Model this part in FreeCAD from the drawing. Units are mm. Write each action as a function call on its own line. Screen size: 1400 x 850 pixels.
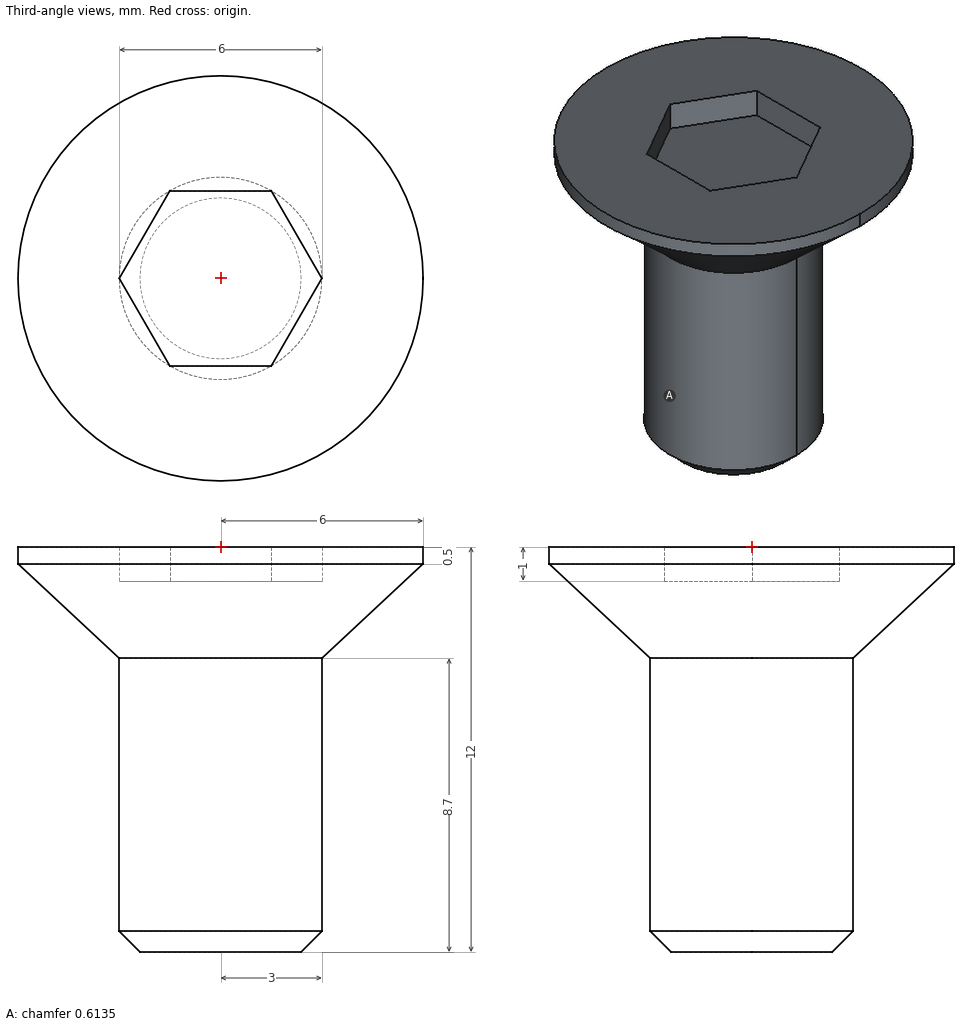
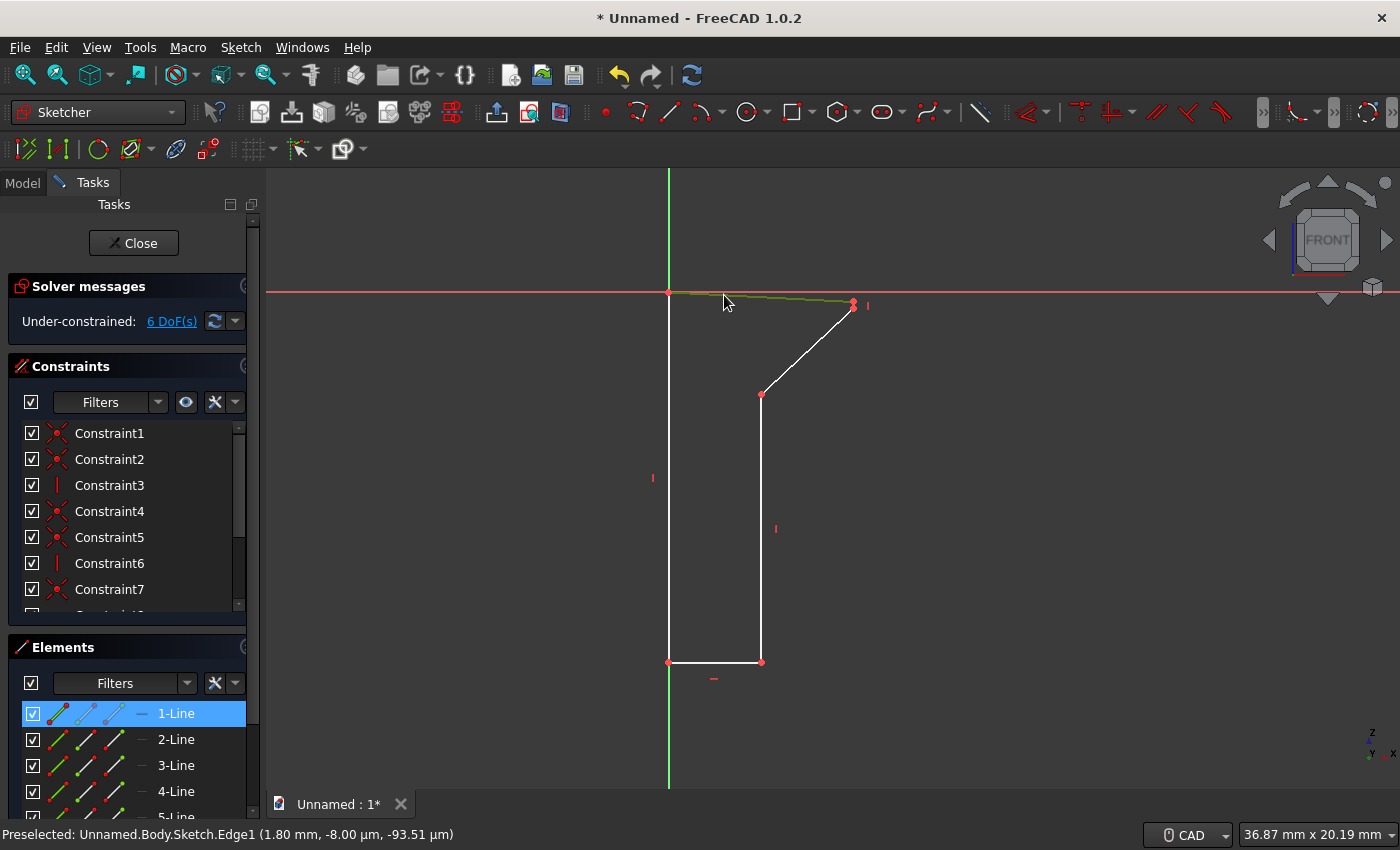
key(h)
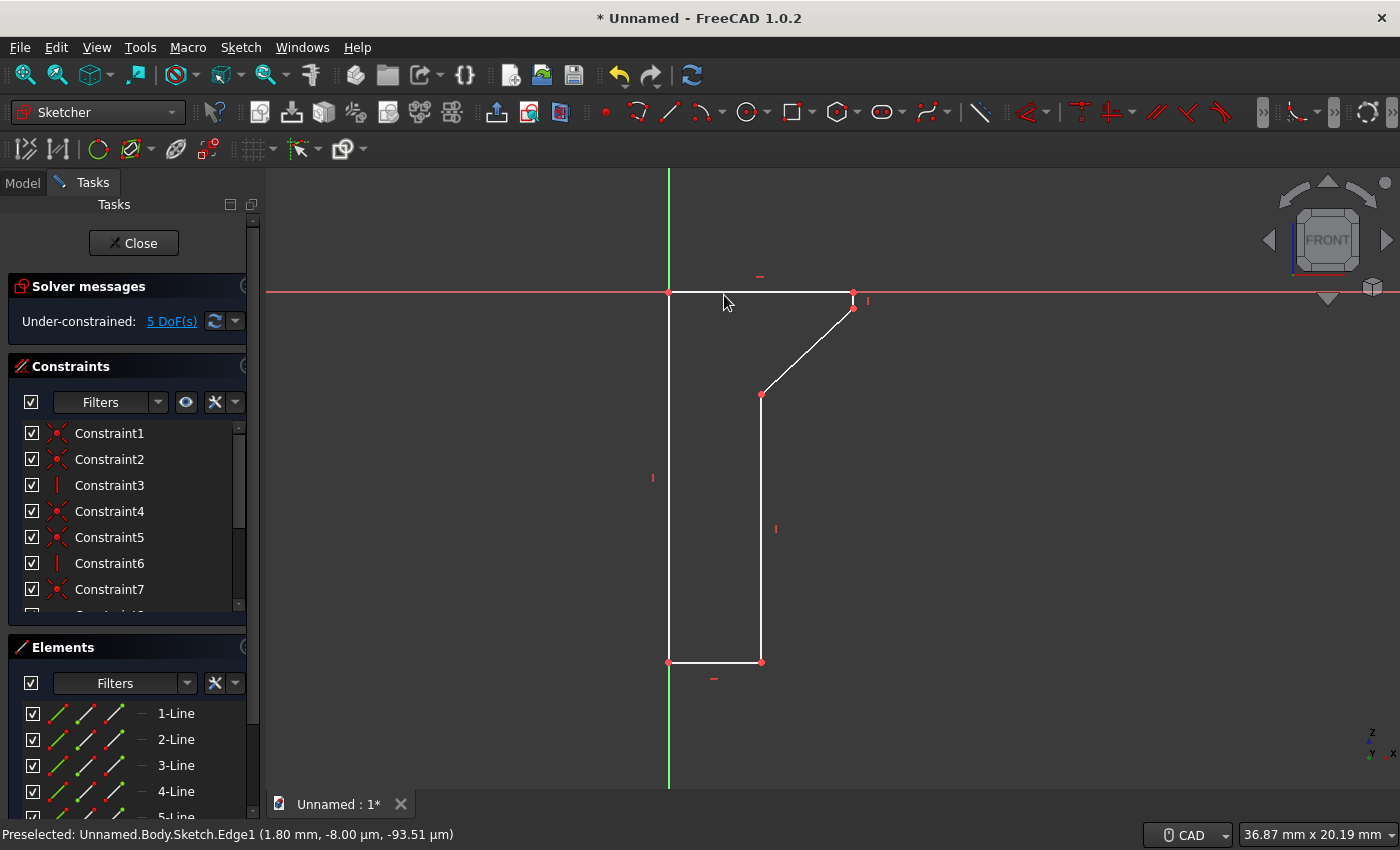
key(d)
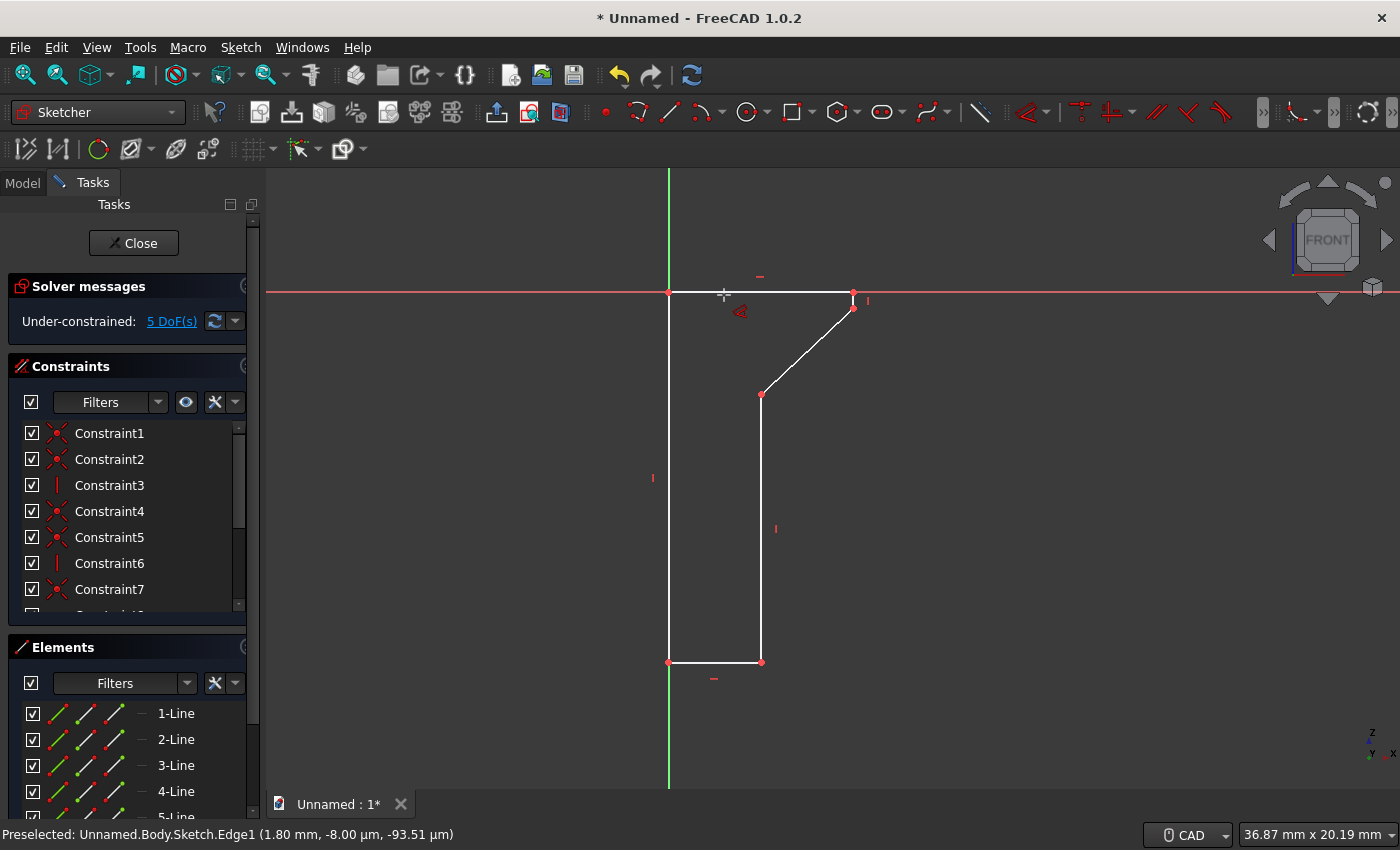
click(724, 292)
click(761, 258)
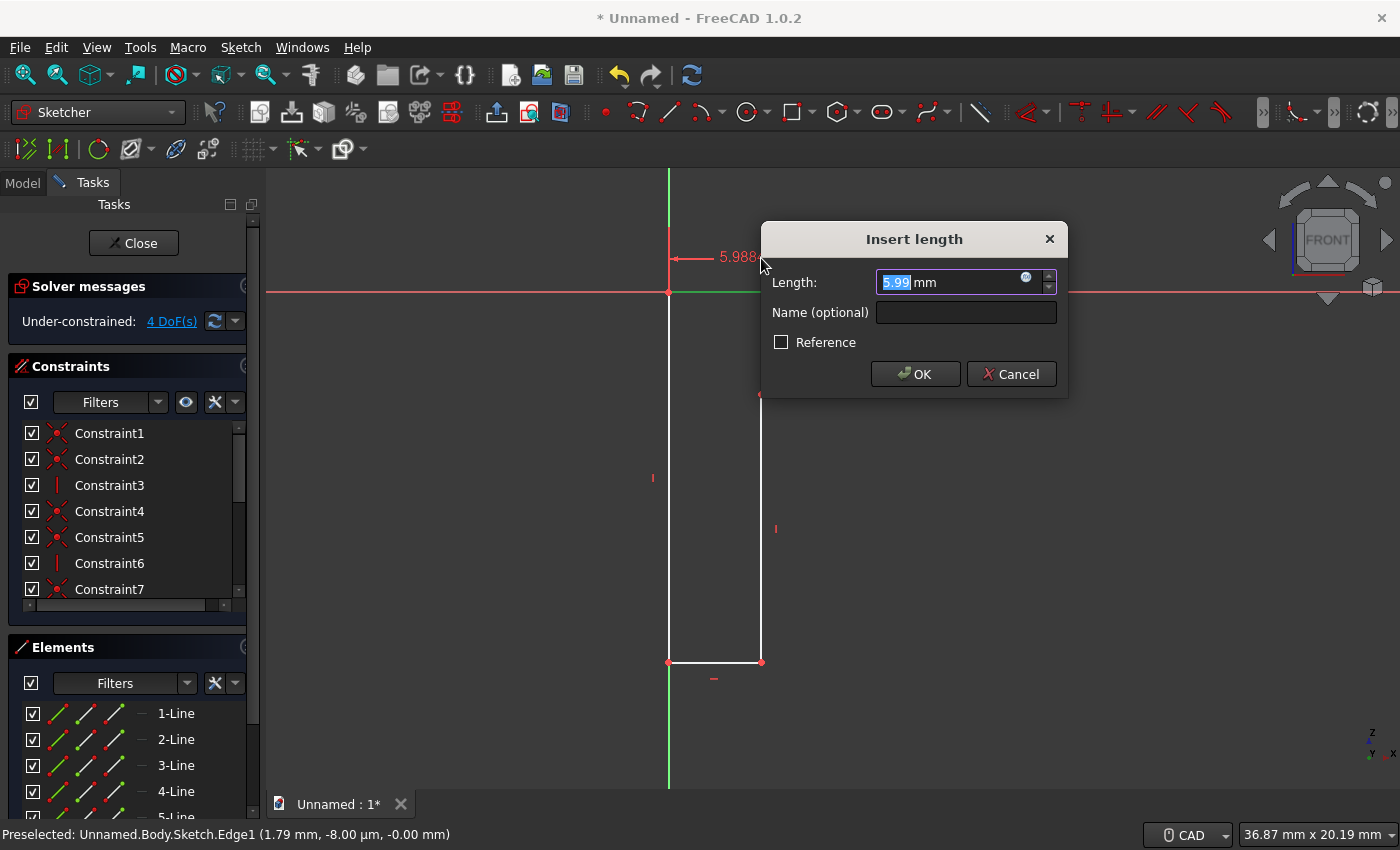
text(6)
key(Return)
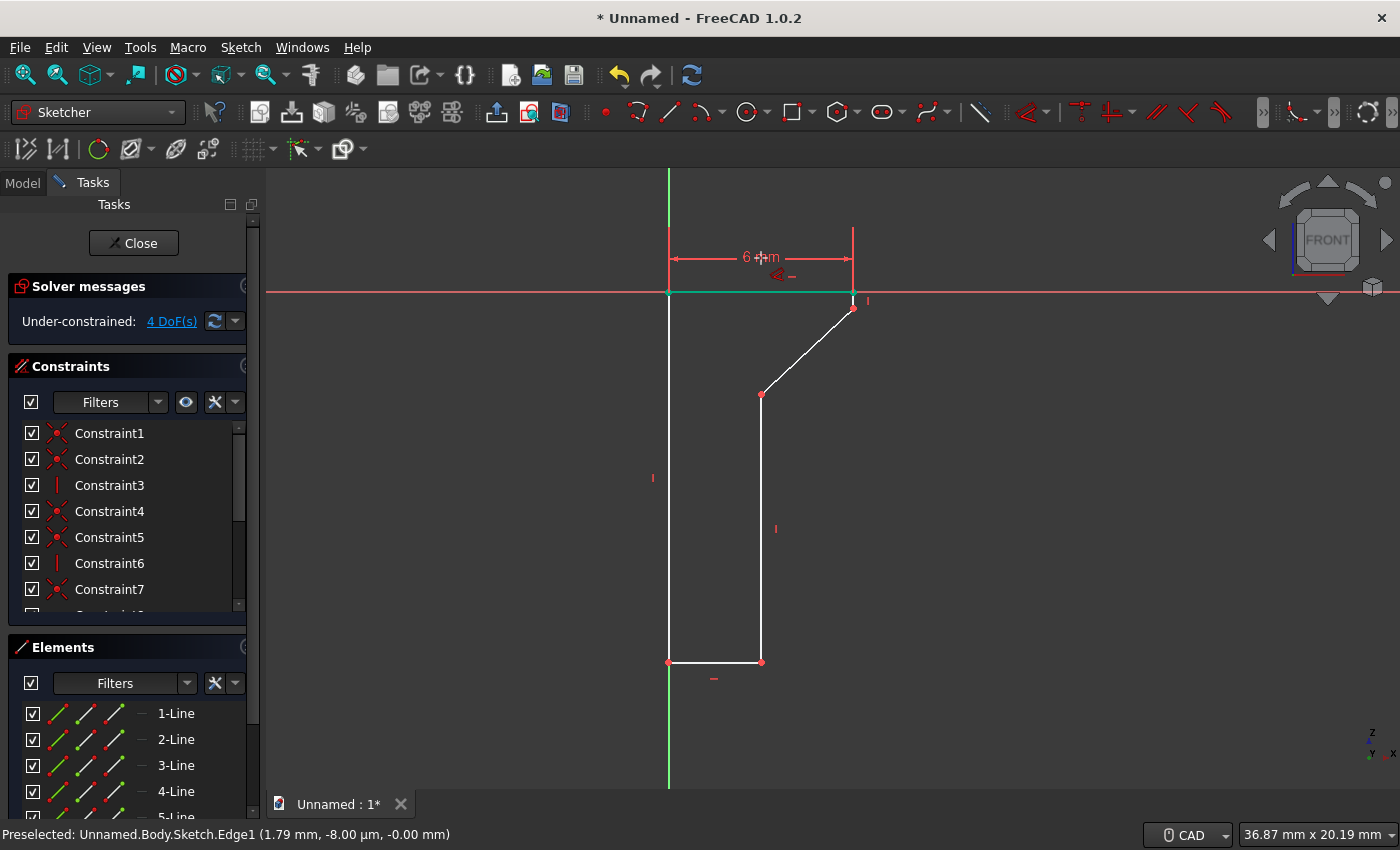
click(733, 663)
click(715, 697)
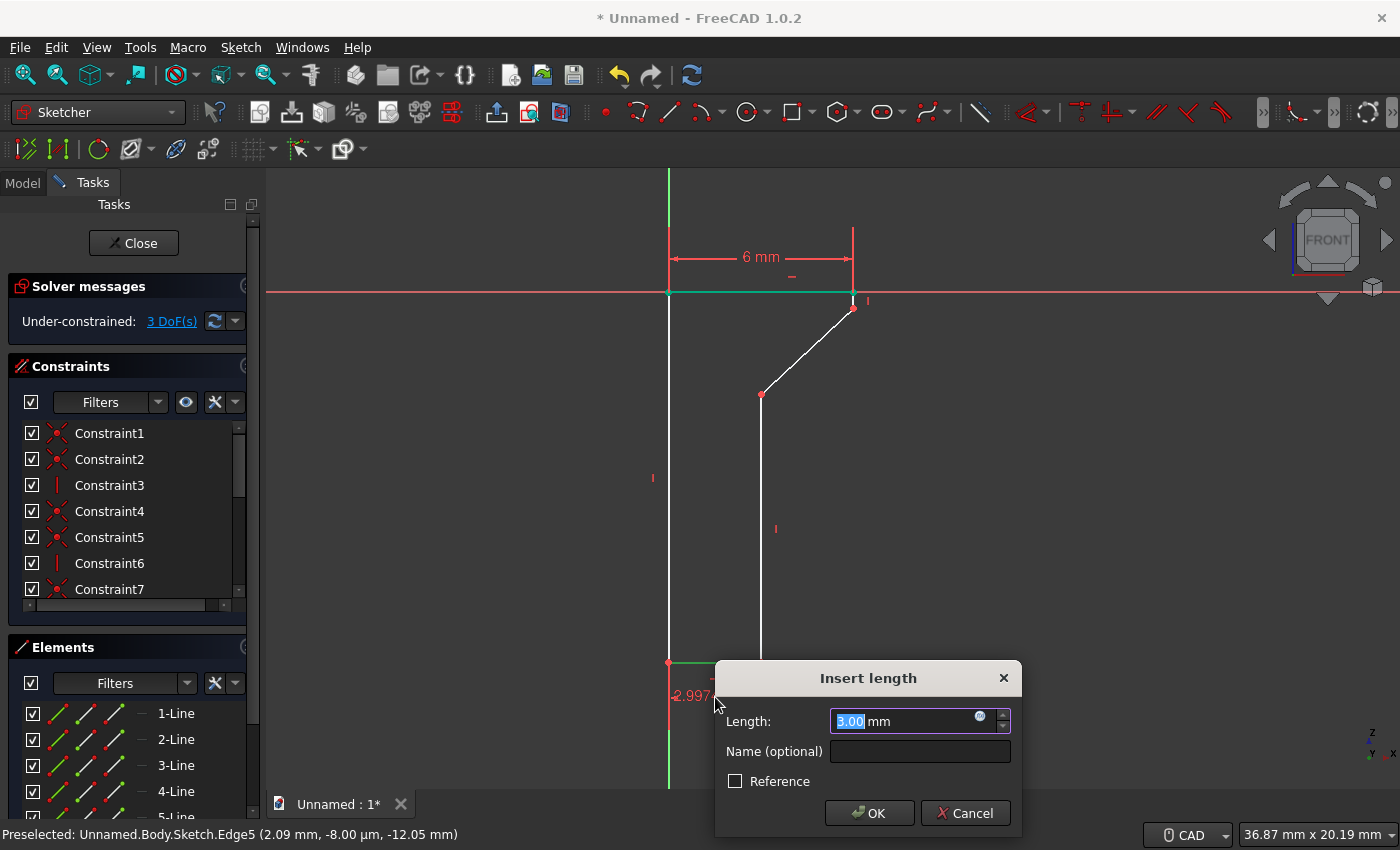
text(3)
key(Return)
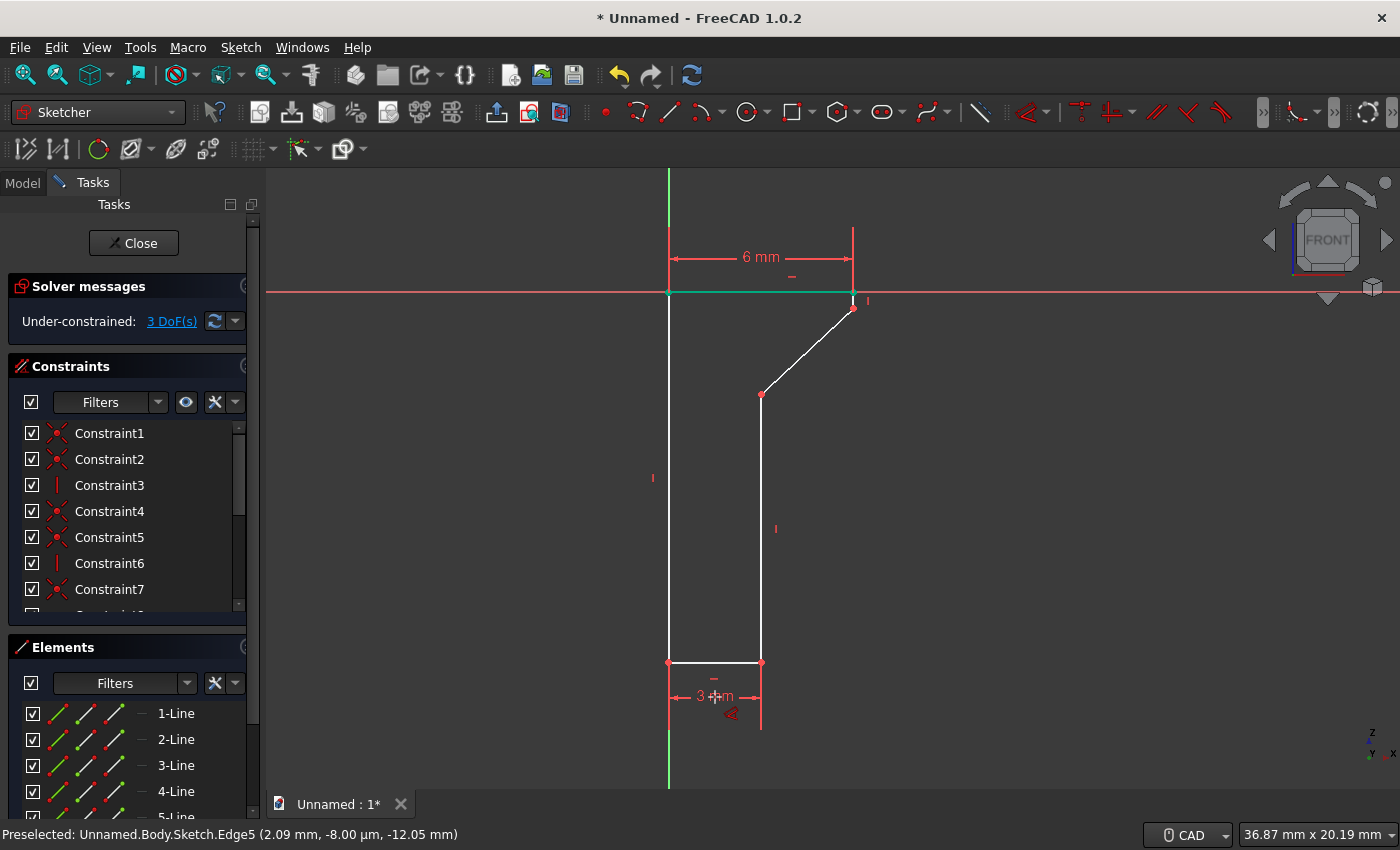
click(669, 552)
click(635, 478)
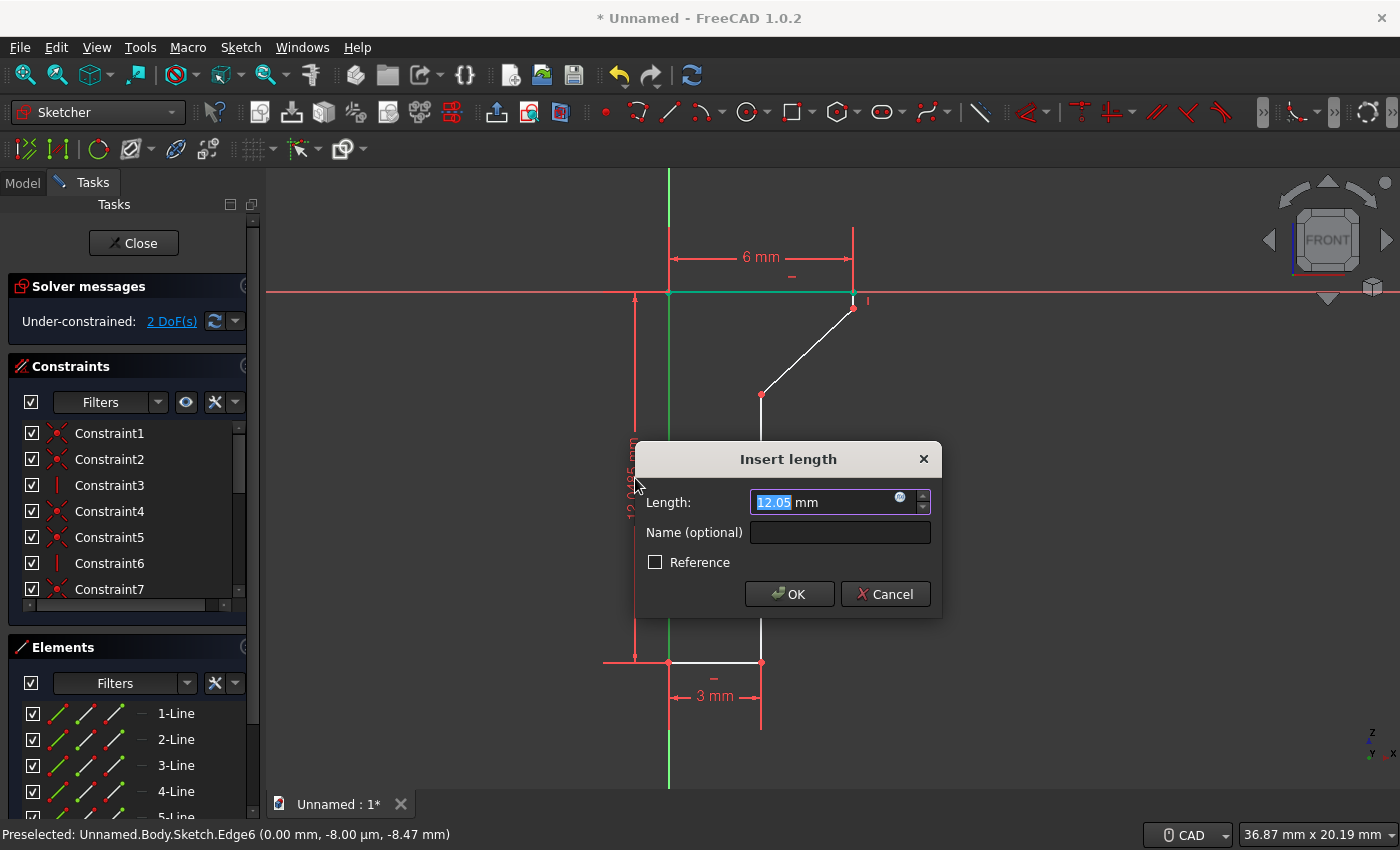
text(12)
key(Return)